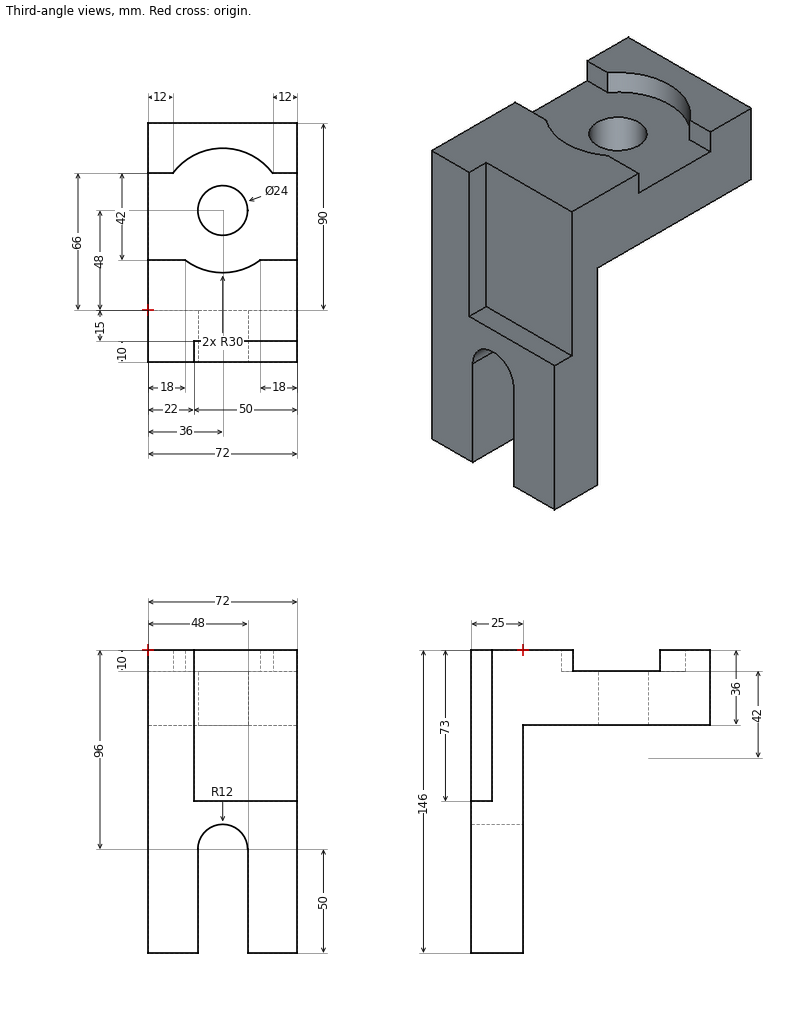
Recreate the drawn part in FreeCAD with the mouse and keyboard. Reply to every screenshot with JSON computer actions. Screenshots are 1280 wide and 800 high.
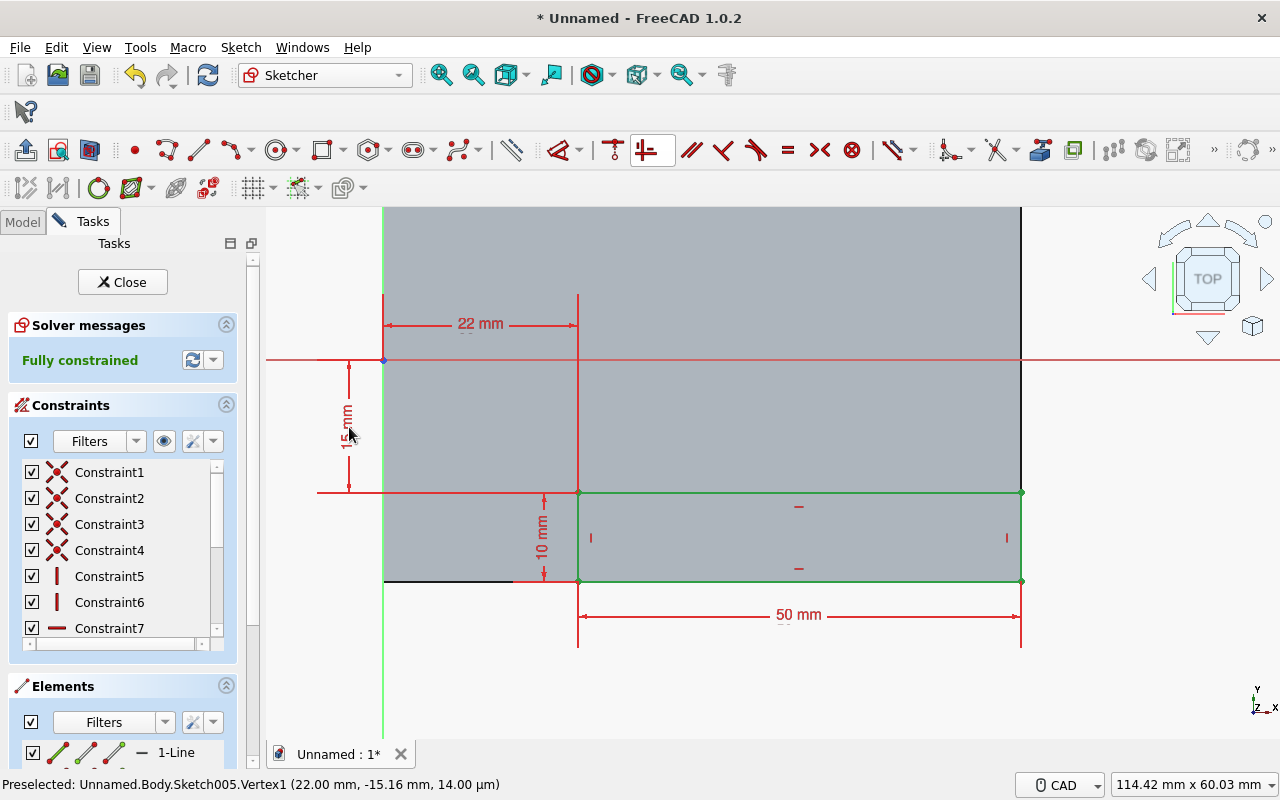
{"action": "left_click", "coordinate": [123, 282]}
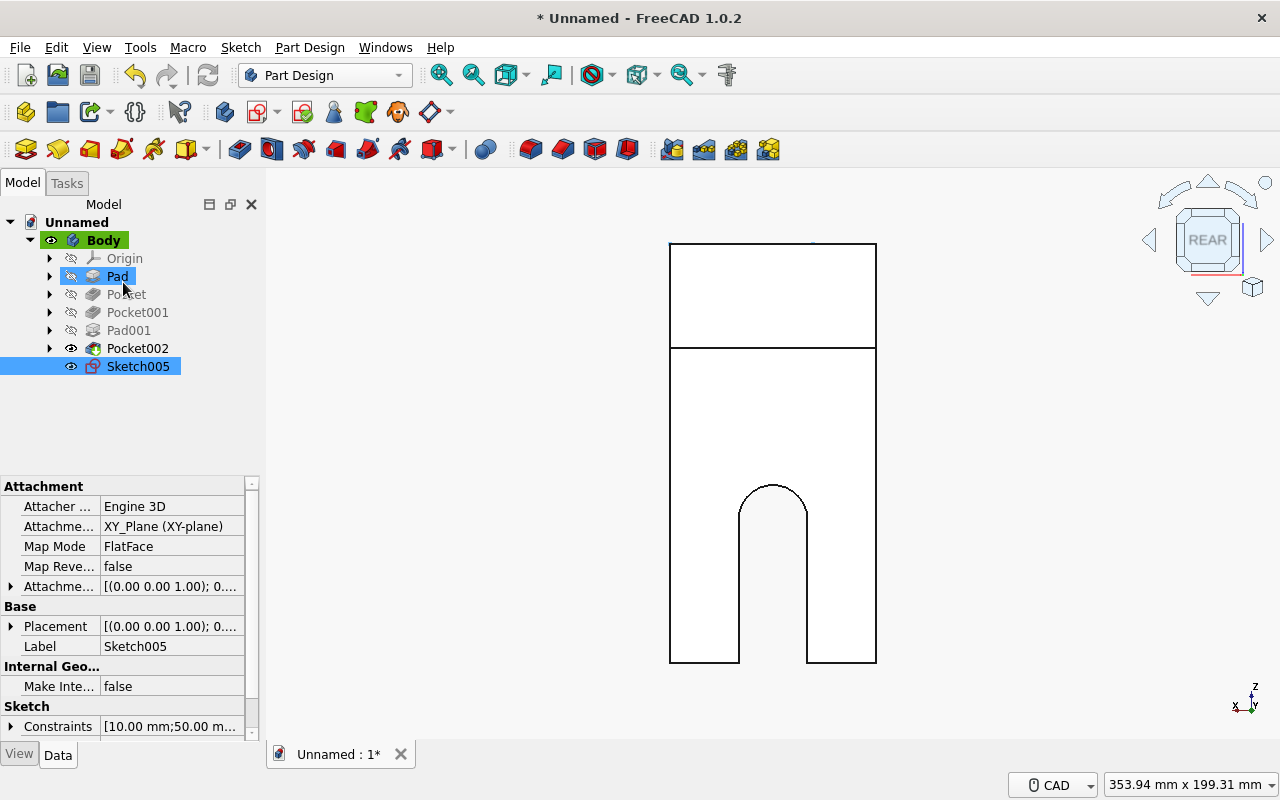
{"action": "left_click", "coordinate": [240, 150]}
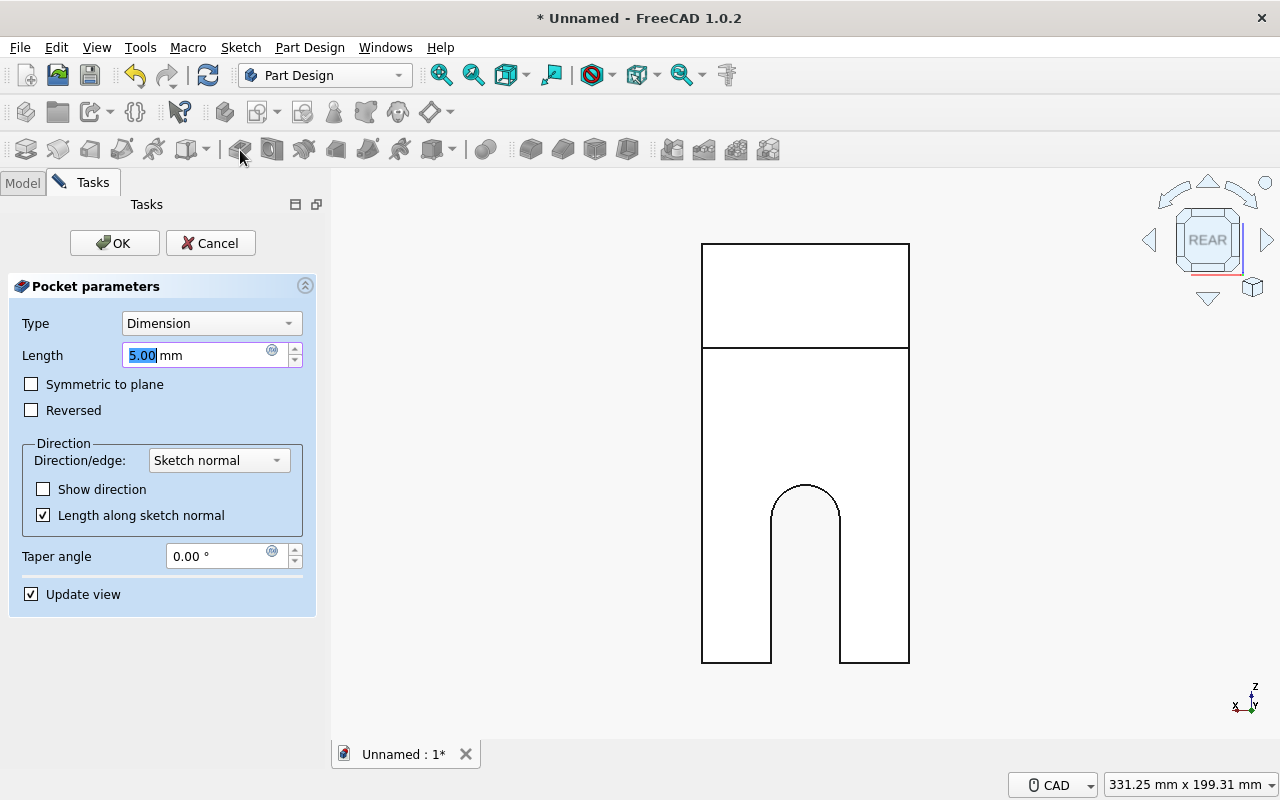
{"action": "type", "text": "73"}
{"action": "key", "text": "Tab"}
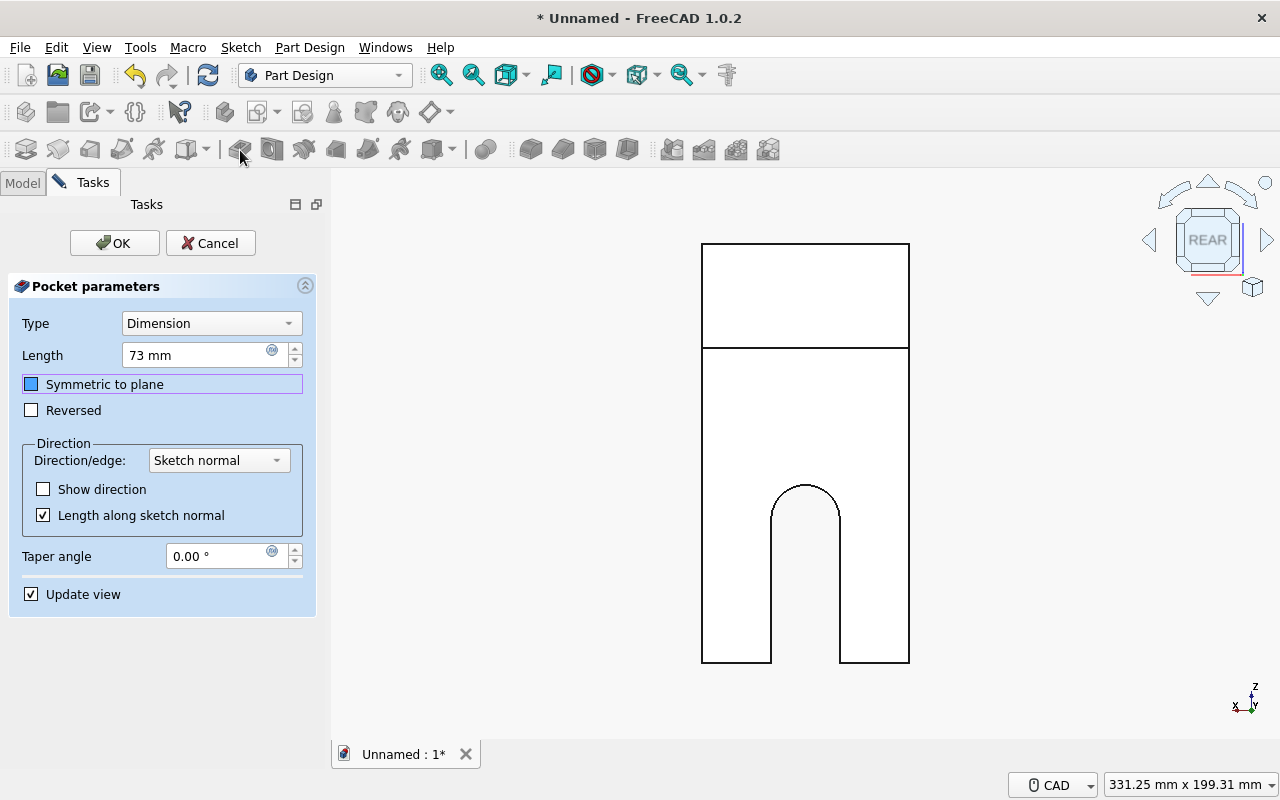
{"action": "left_click", "coordinate": [115, 243]}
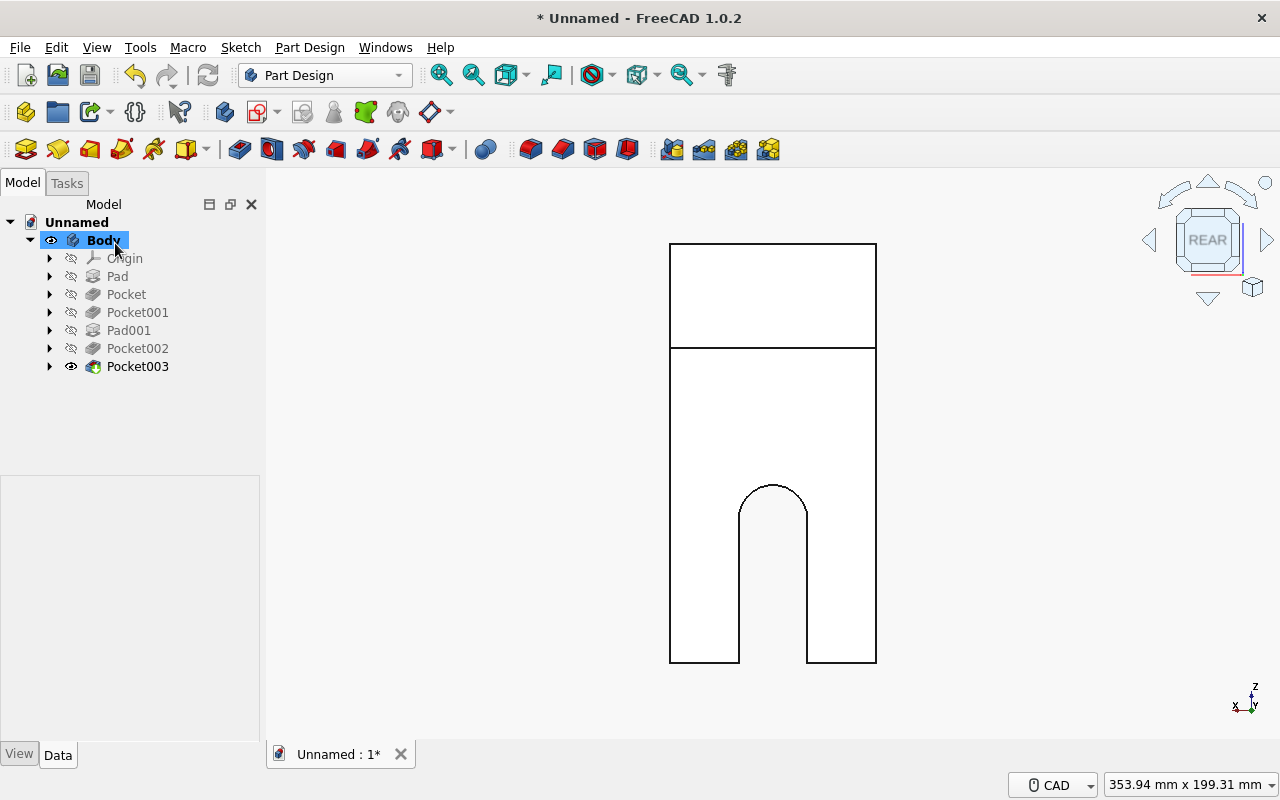
{"action": "key", "text": "0"}